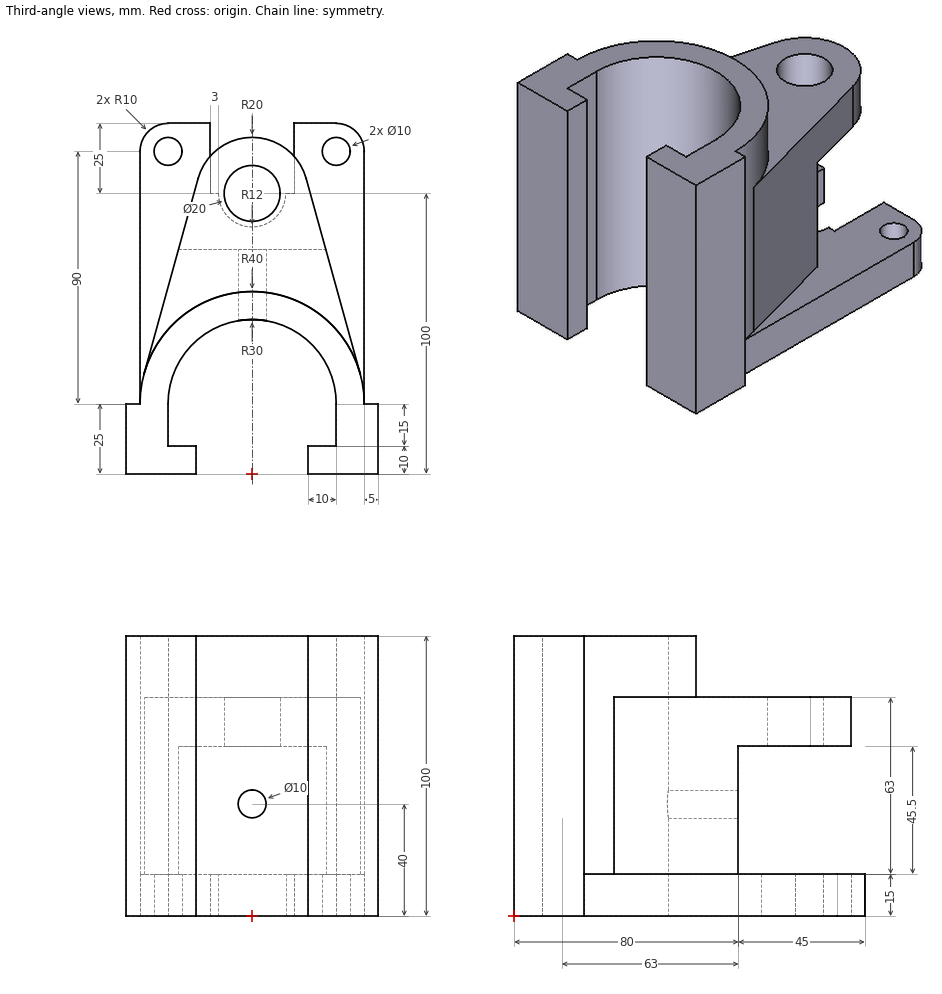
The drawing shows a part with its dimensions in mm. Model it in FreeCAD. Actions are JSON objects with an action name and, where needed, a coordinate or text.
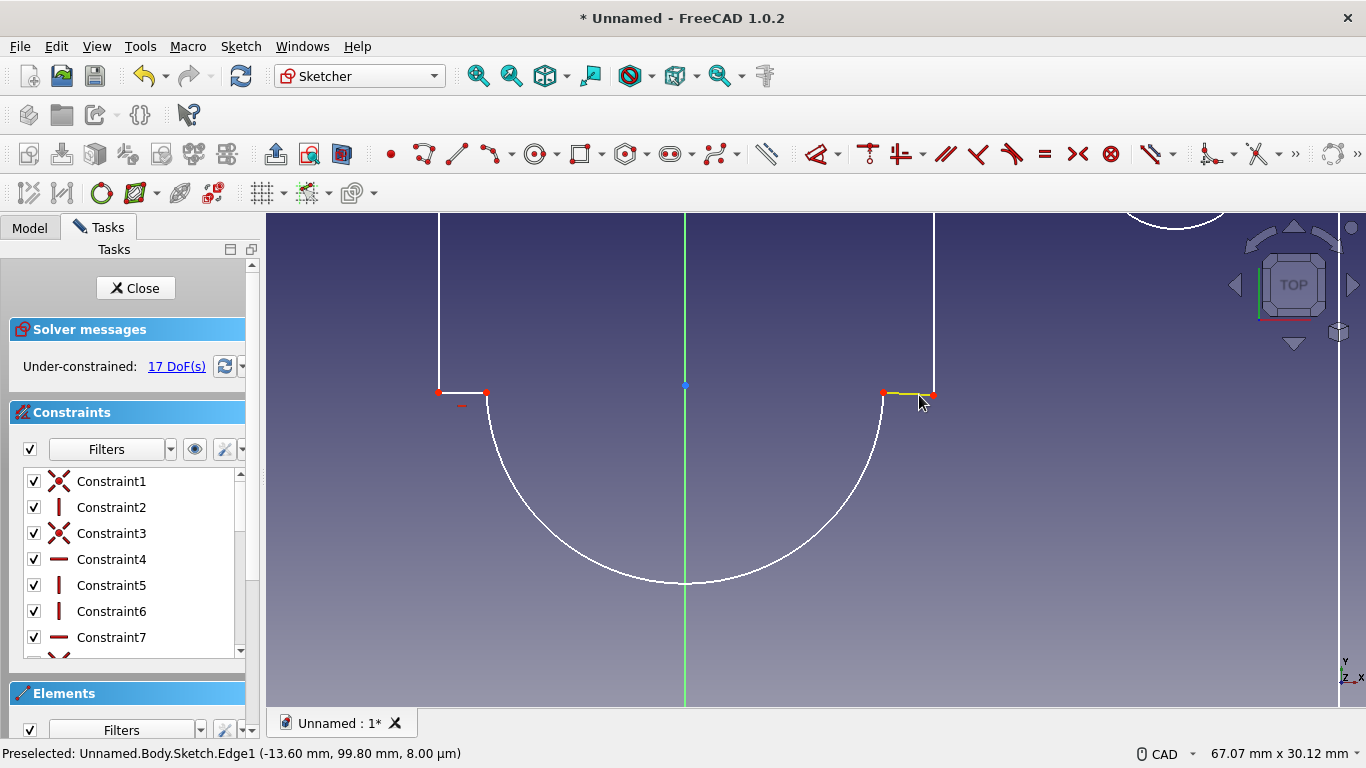
{"action": "left_click", "coordinate": [919, 394]}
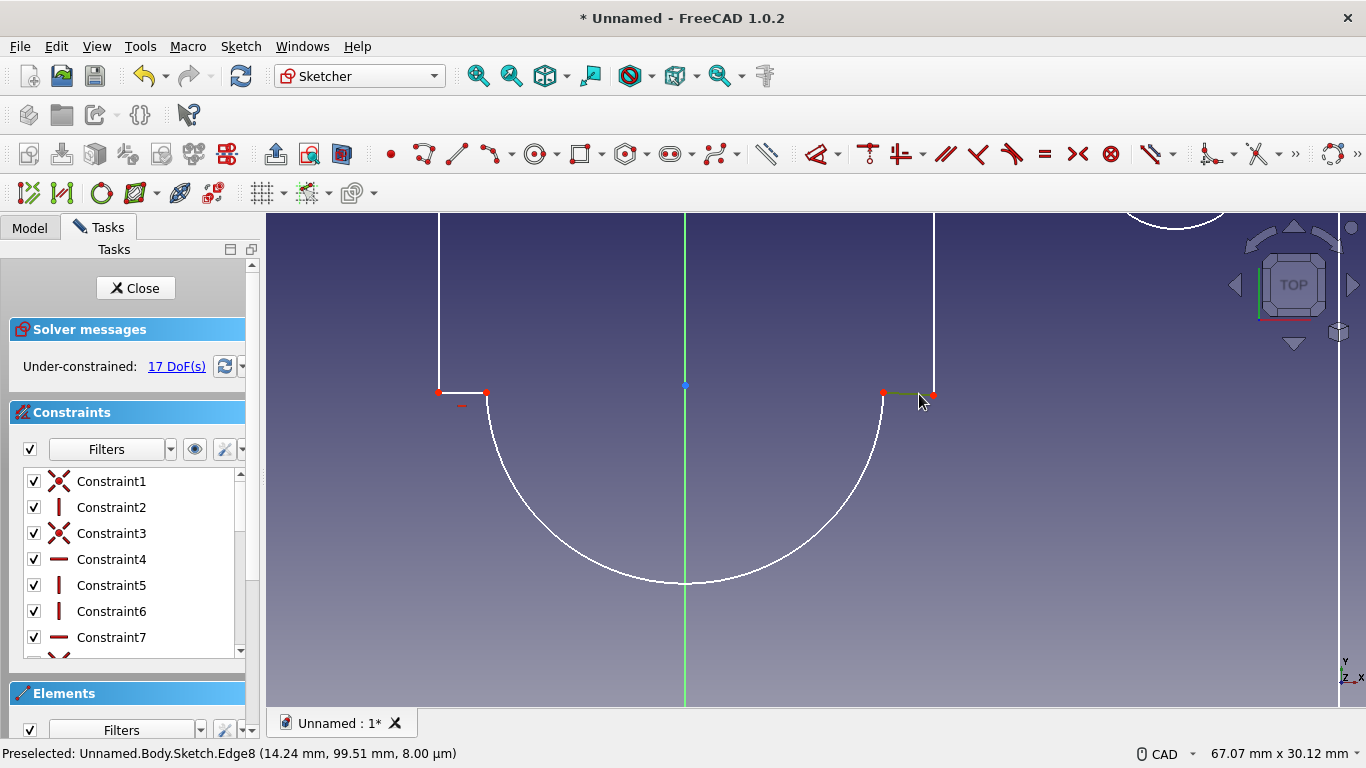
{"action": "key", "text": "h"}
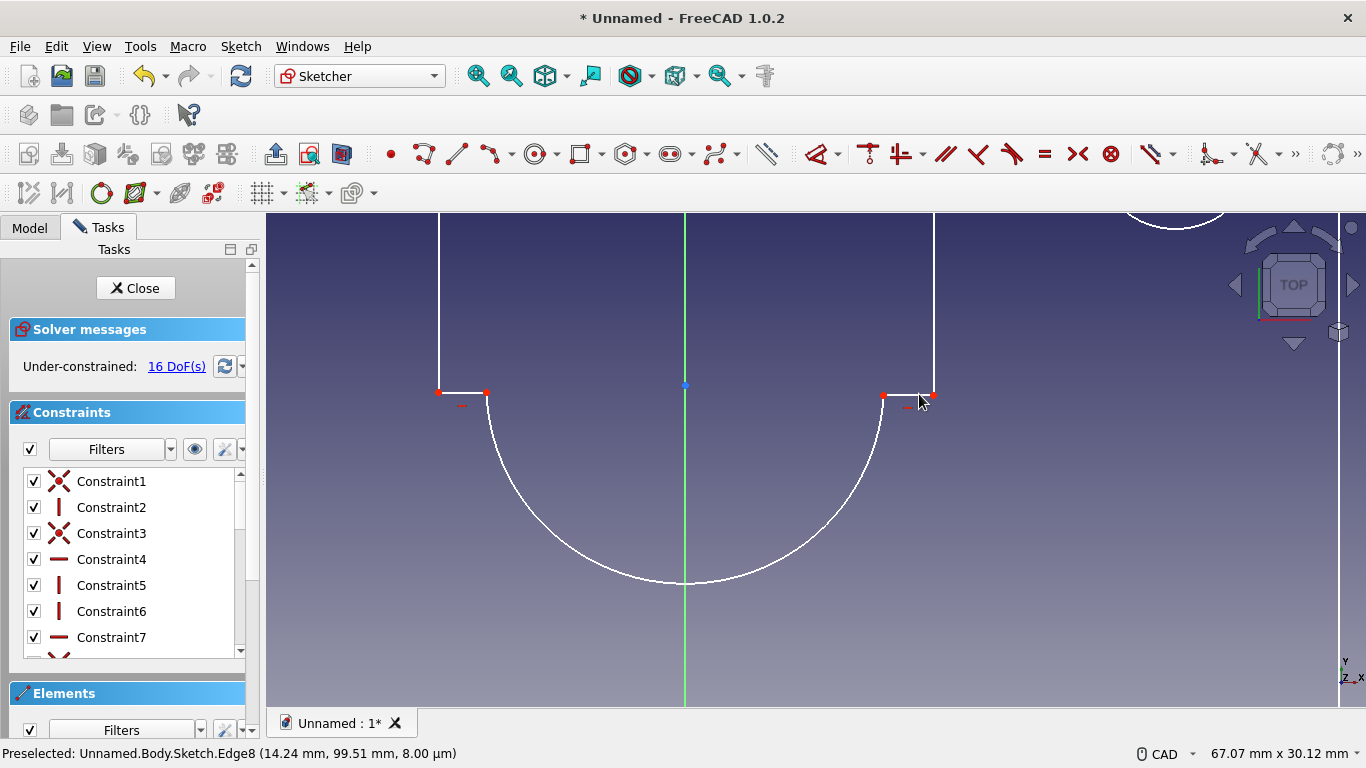
{"action": "scroll", "coordinate": [760, 353], "scroll_direction": "down", "scroll_amount": 9}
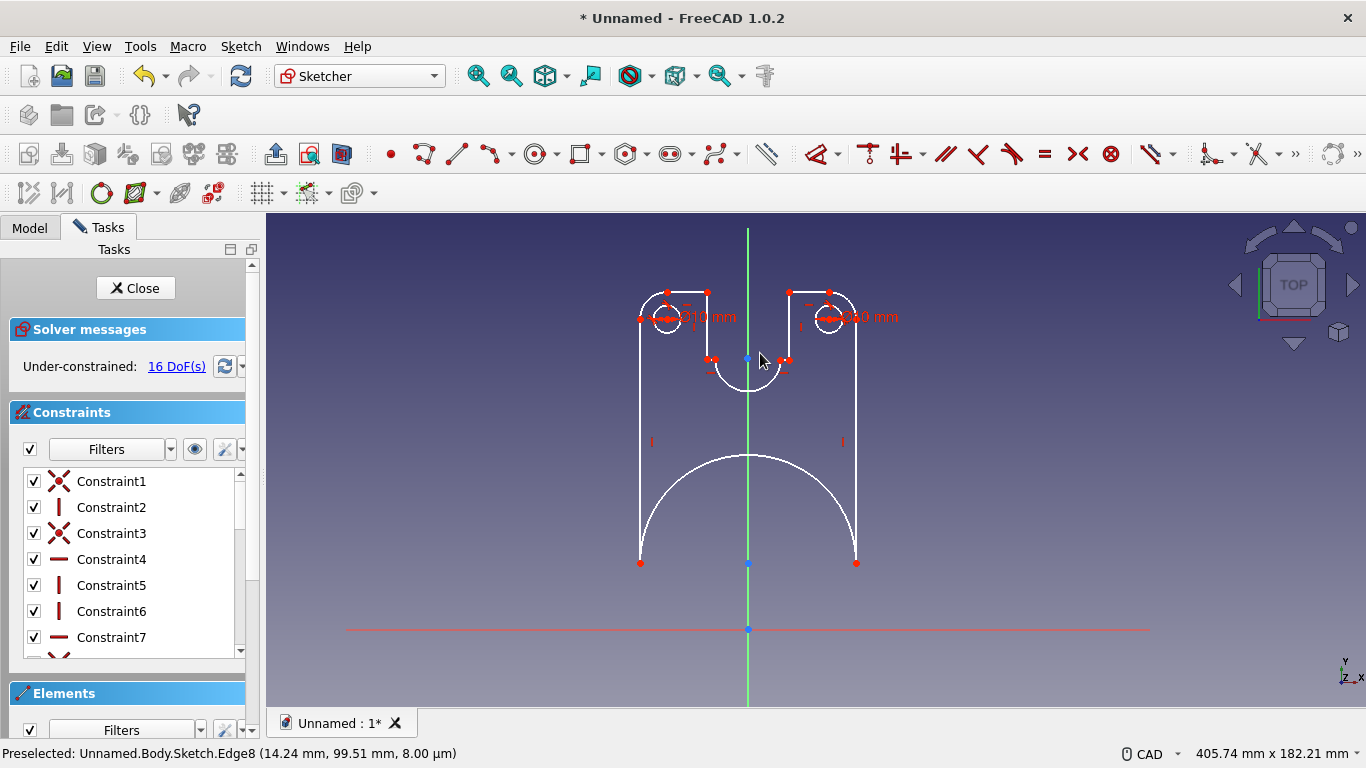
{"action": "left_click", "coordinate": [655, 295]}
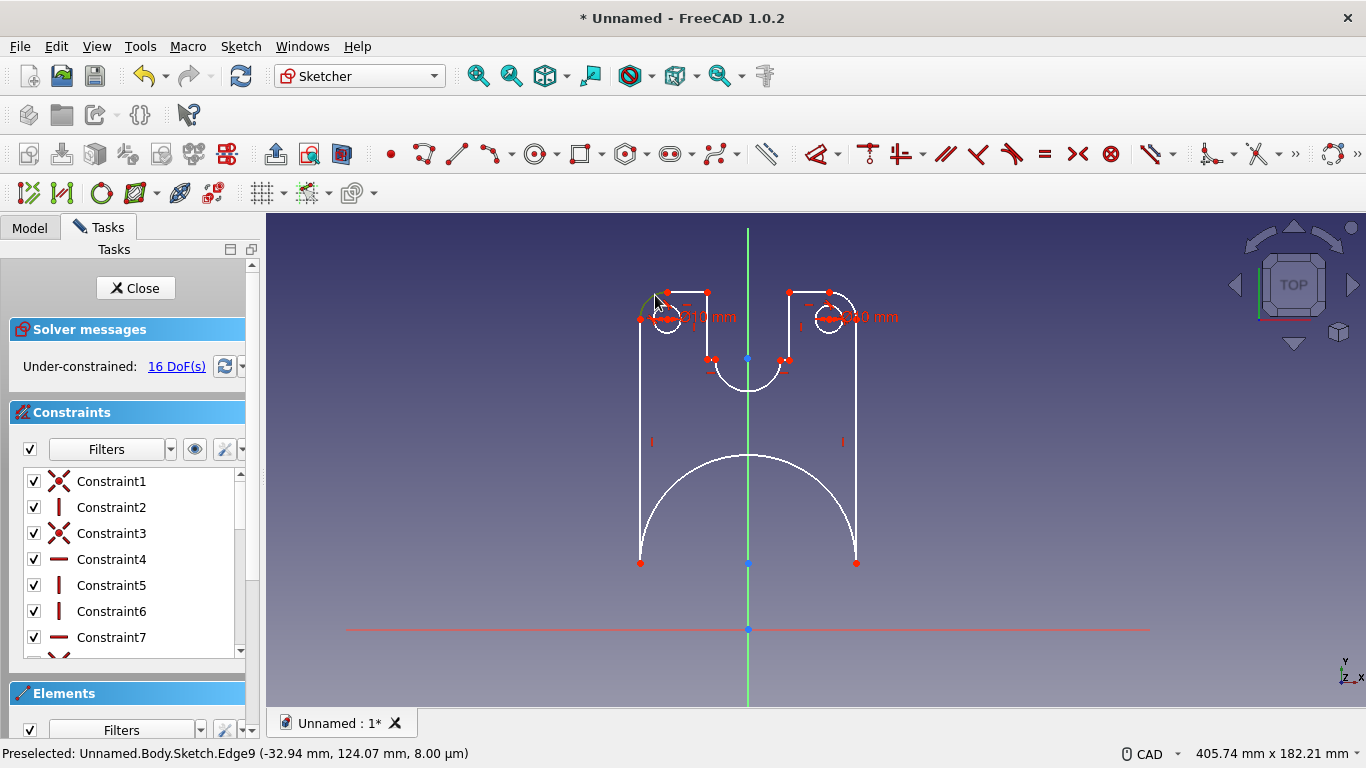
{"action": "left_click", "coordinate": [853, 307]}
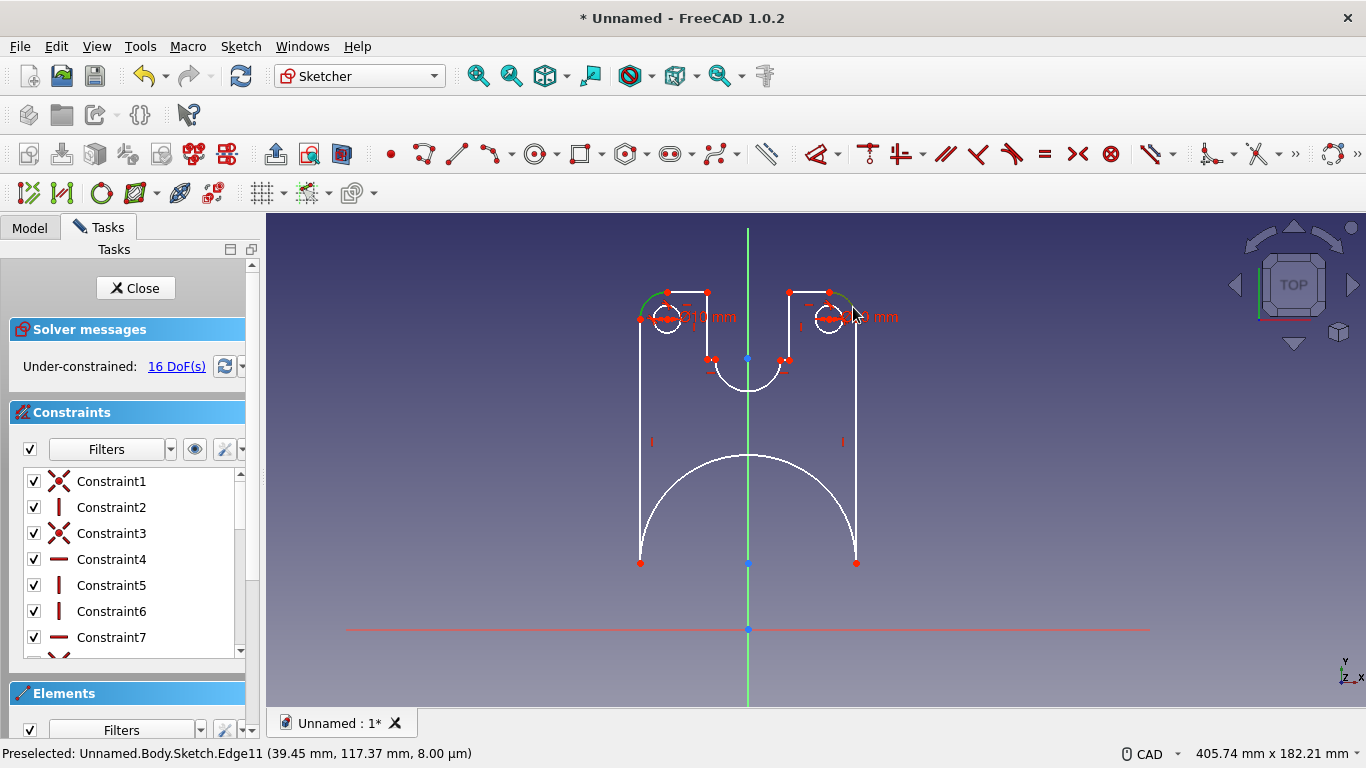
{"action": "key", "text": "e"}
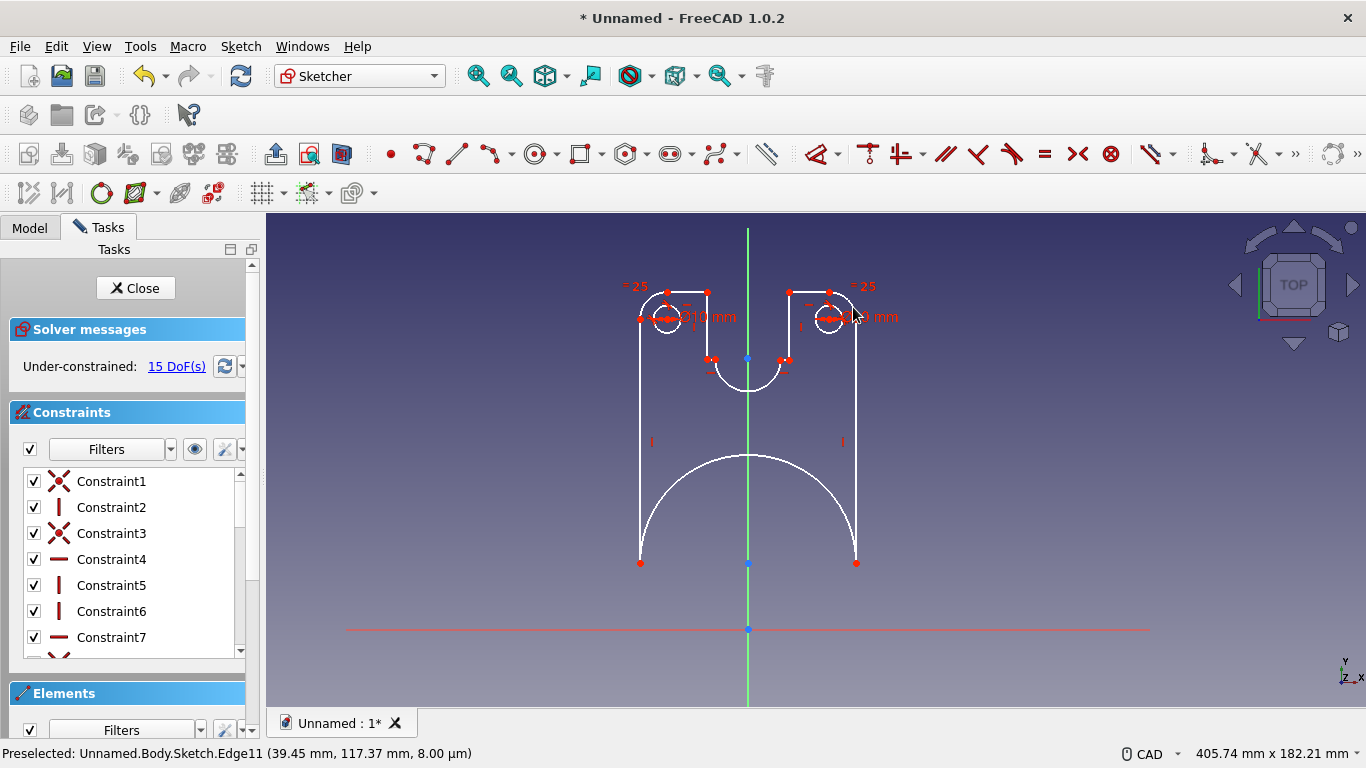
{"action": "left_click", "coordinate": [748, 563]}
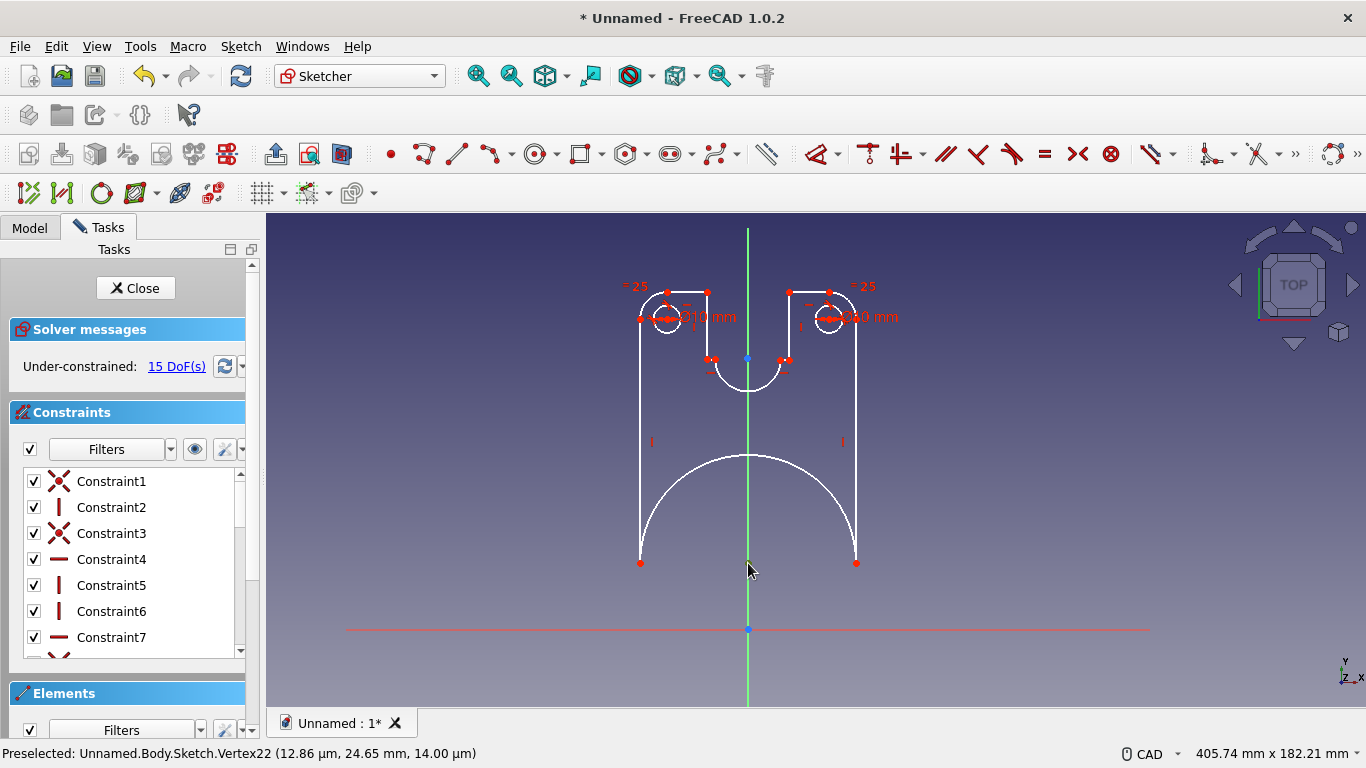
{"action": "left_click", "coordinate": [748, 585]}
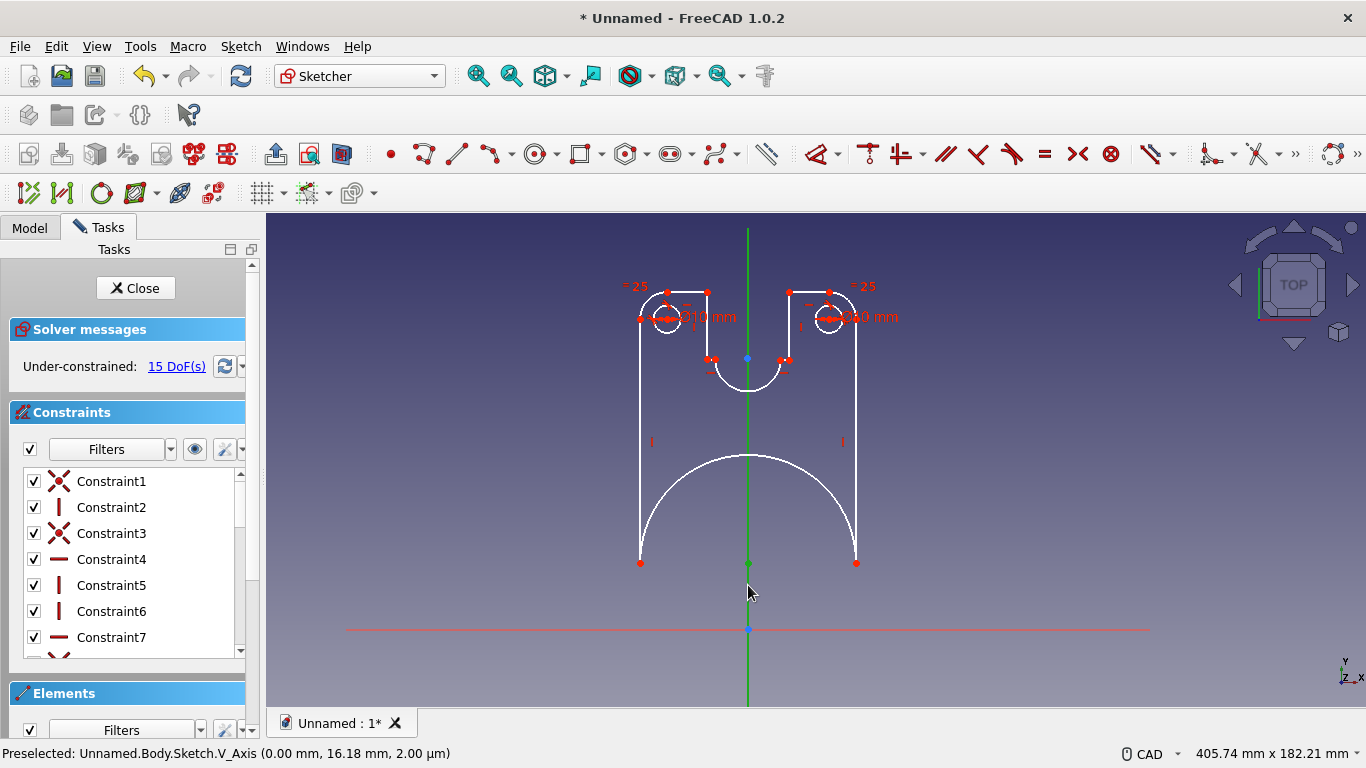
{"action": "left_click", "coordinate": [868, 154]}